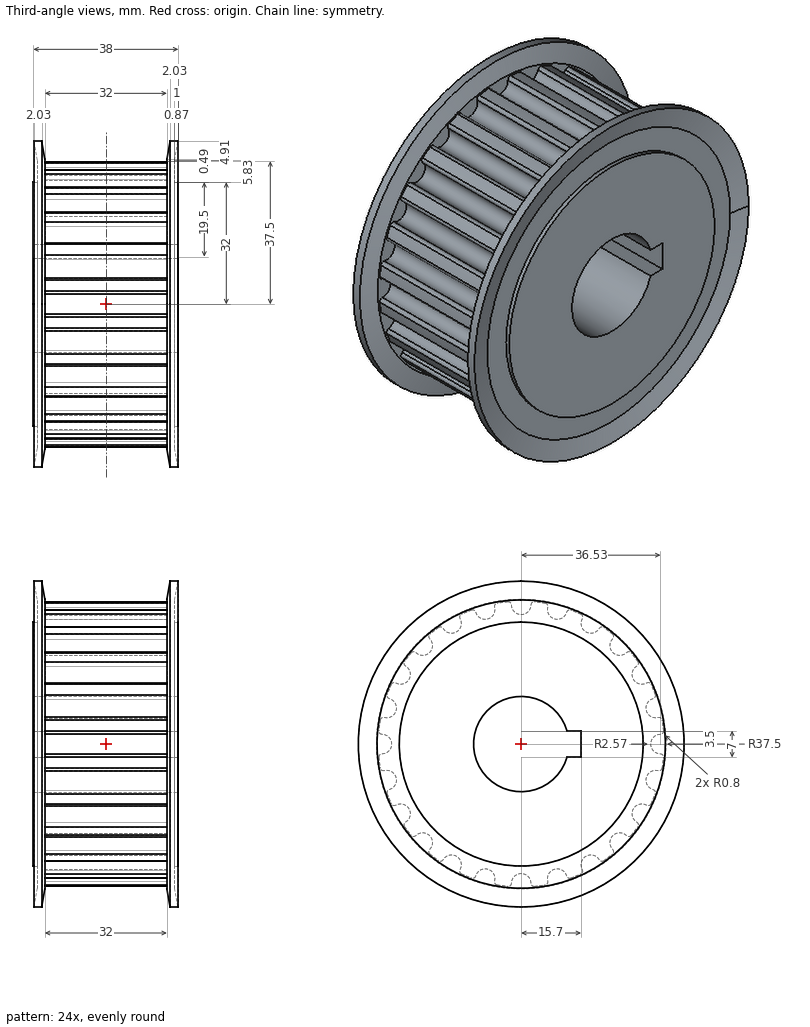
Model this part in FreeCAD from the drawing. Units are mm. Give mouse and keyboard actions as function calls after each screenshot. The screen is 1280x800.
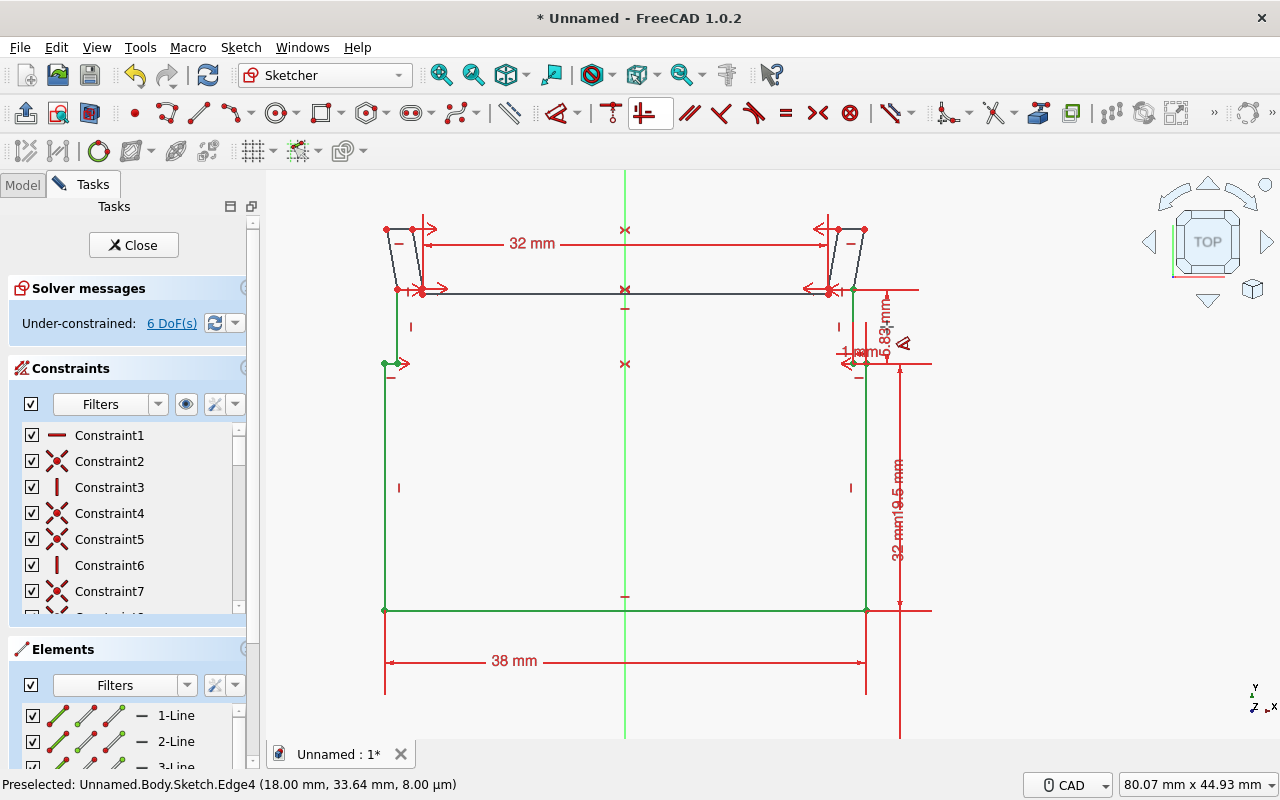
scroll(854, 229, up, 3)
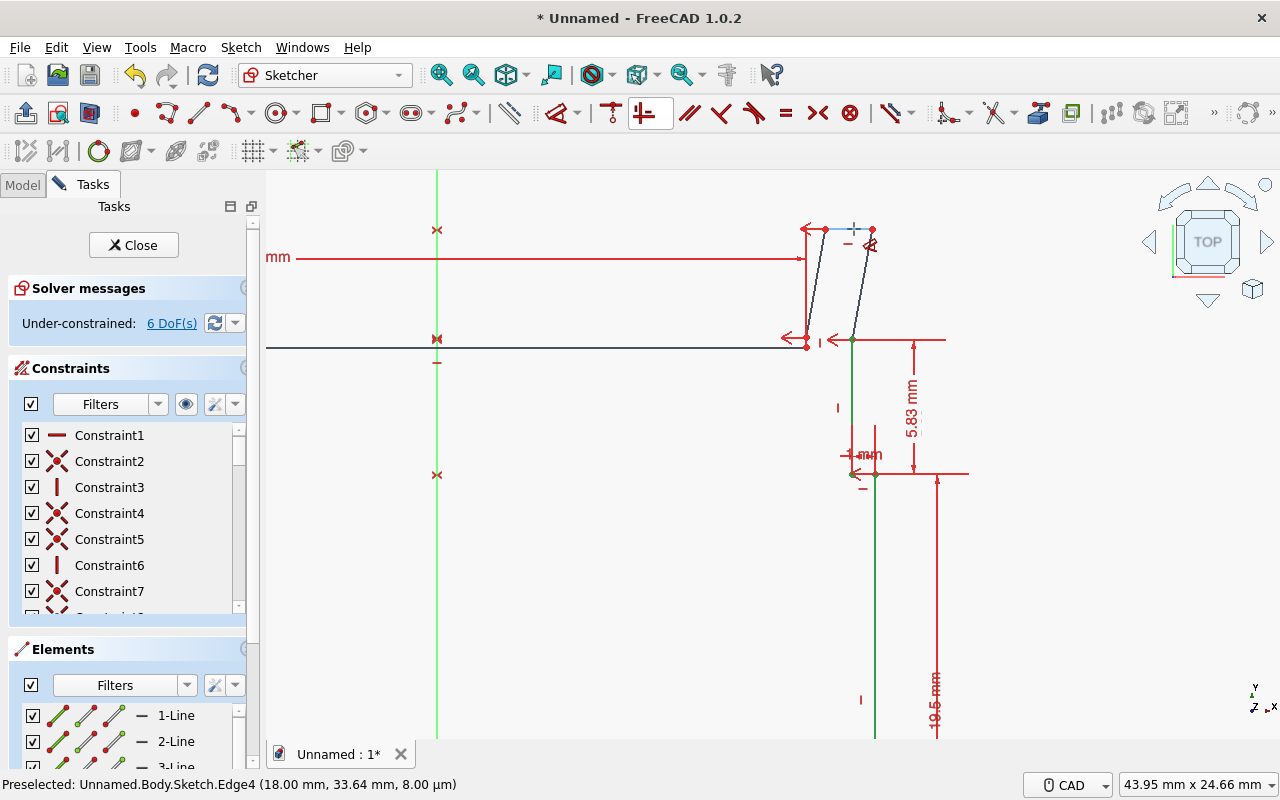
click(854, 229)
click(849, 263)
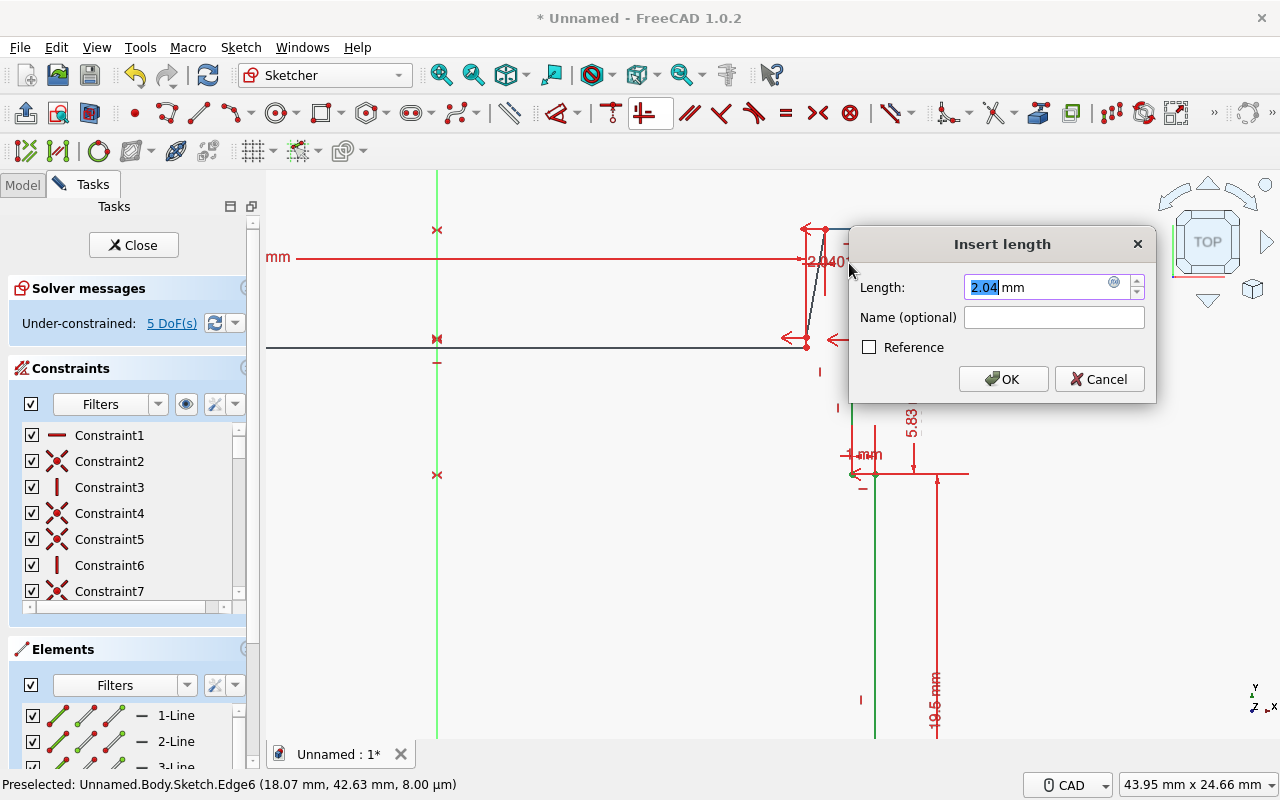
text(2.03)
key(Return)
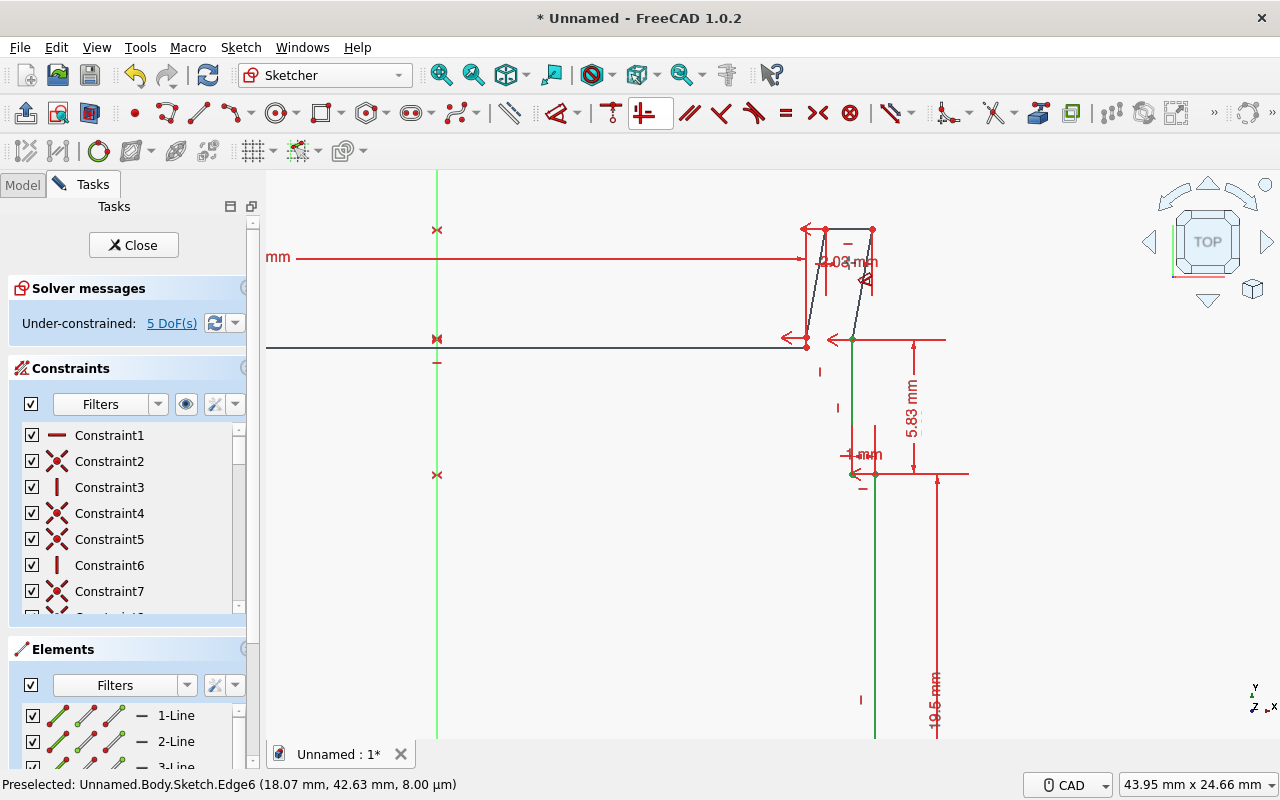
scroll(806, 343, up, 7)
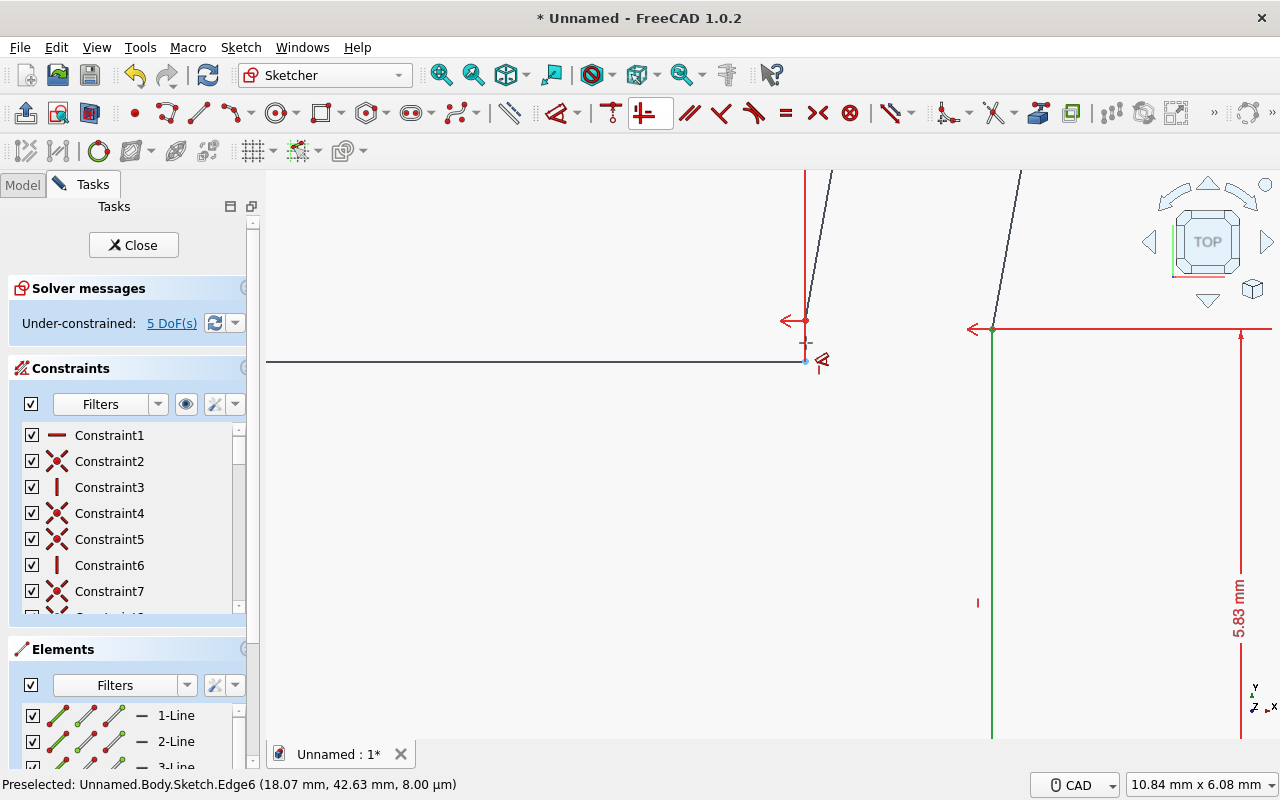
click(805, 341)
click(839, 341)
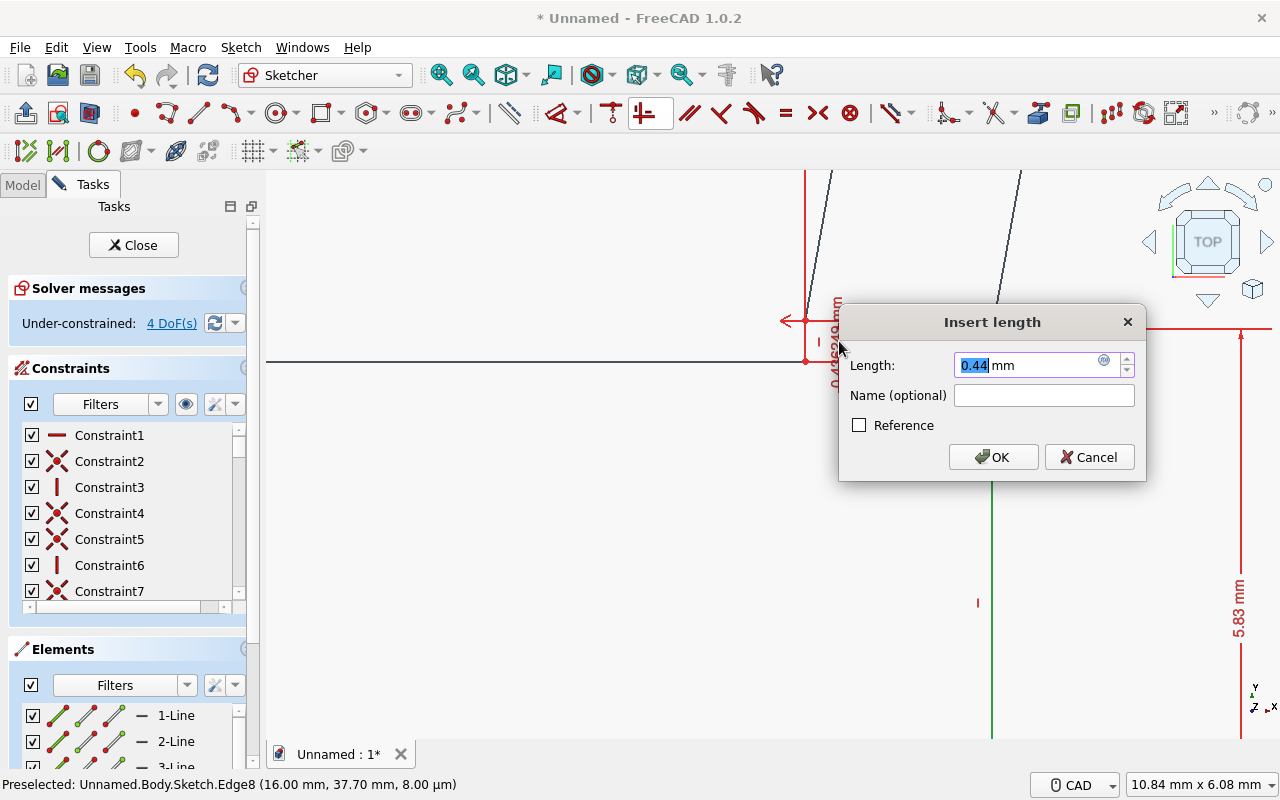
text(0.49)
key(Return)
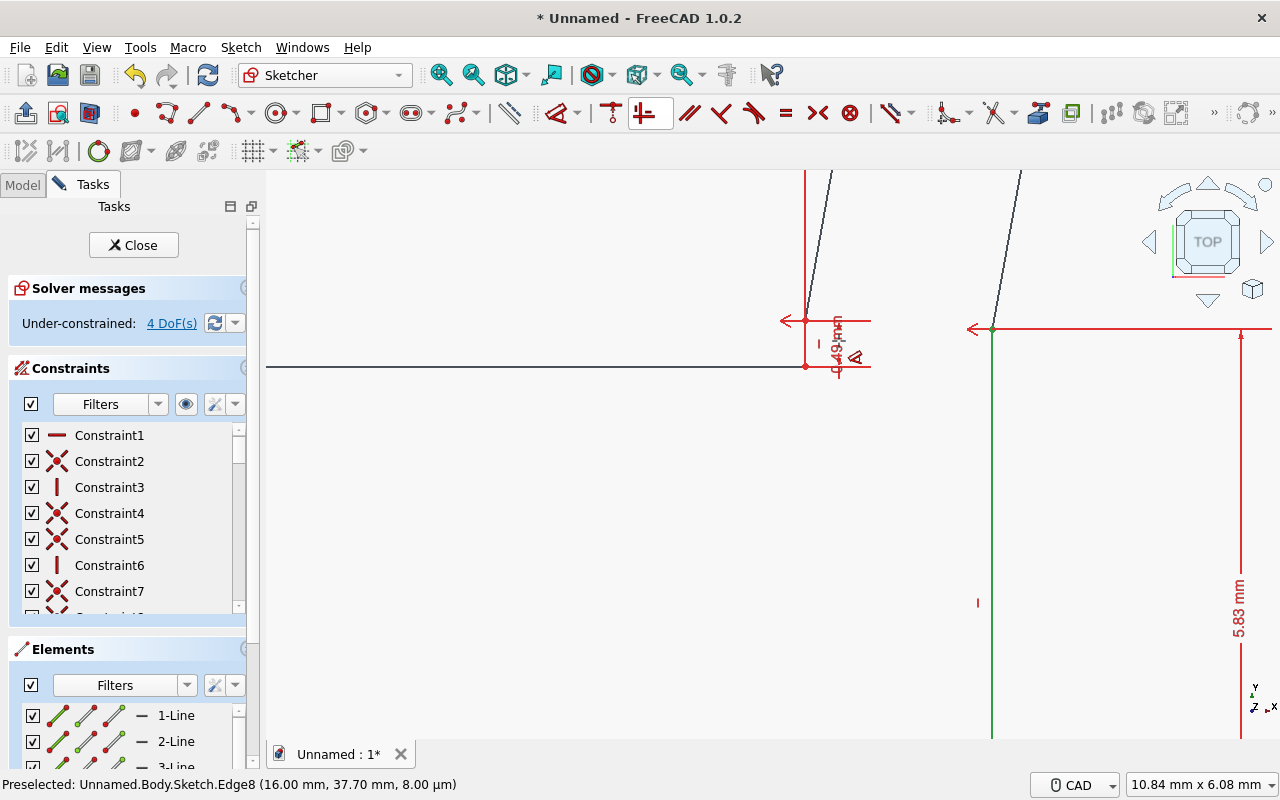
scroll(844, 313, down, 12)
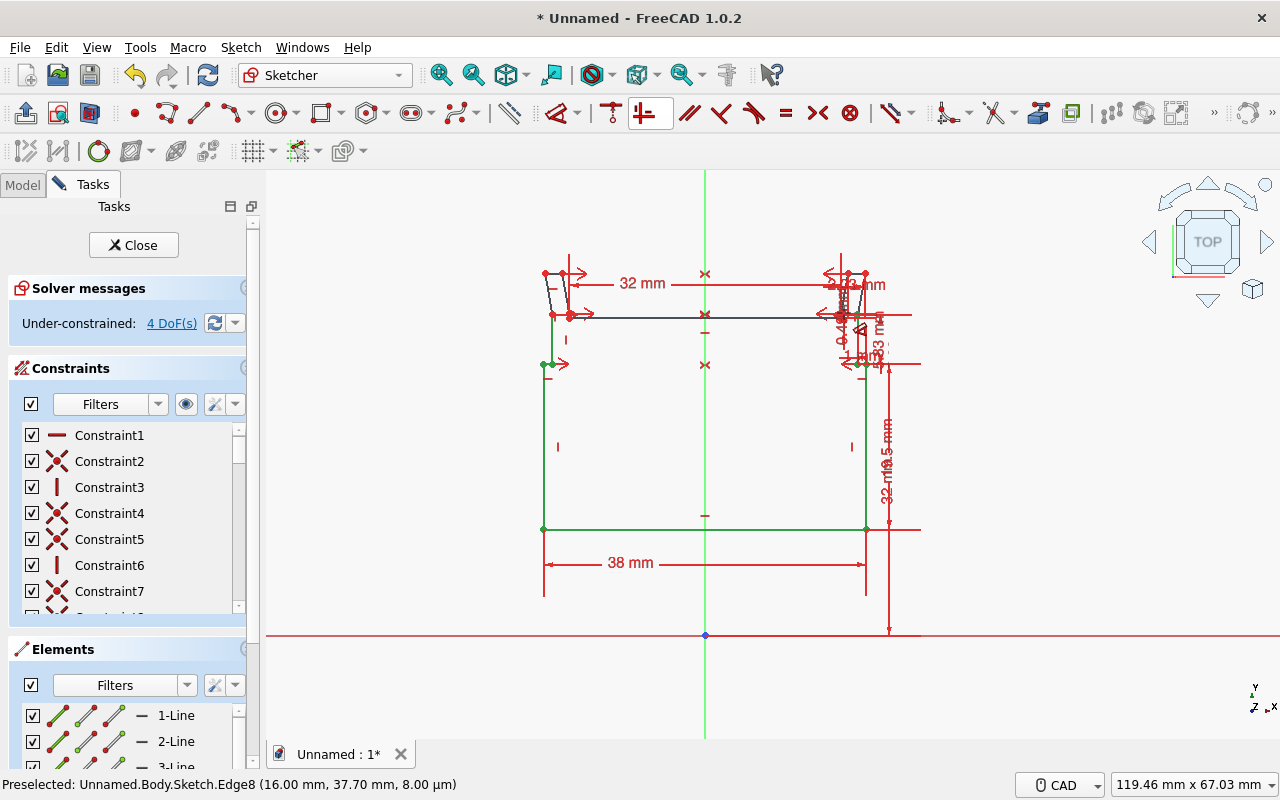
scroll(557, 274, up, 6)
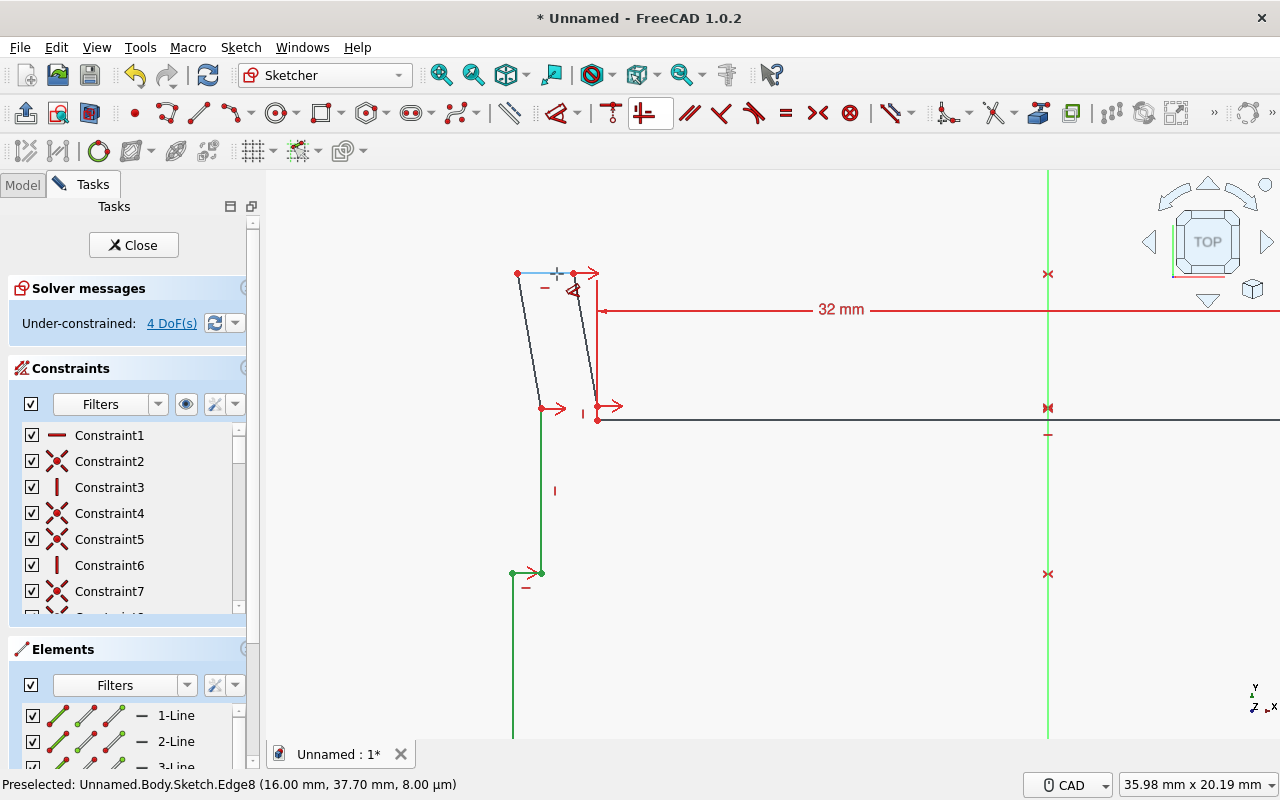
click(557, 273)
click(546, 239)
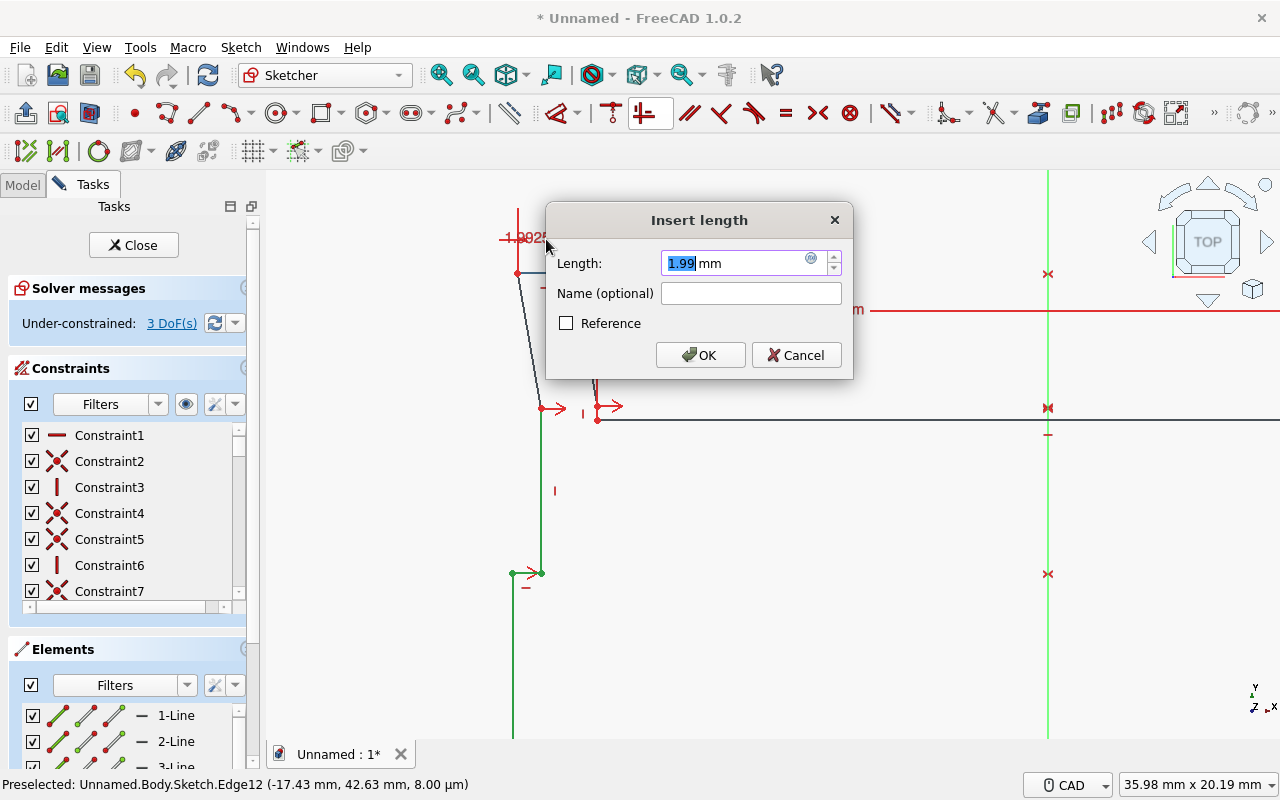
text(2.03)
key(Return)